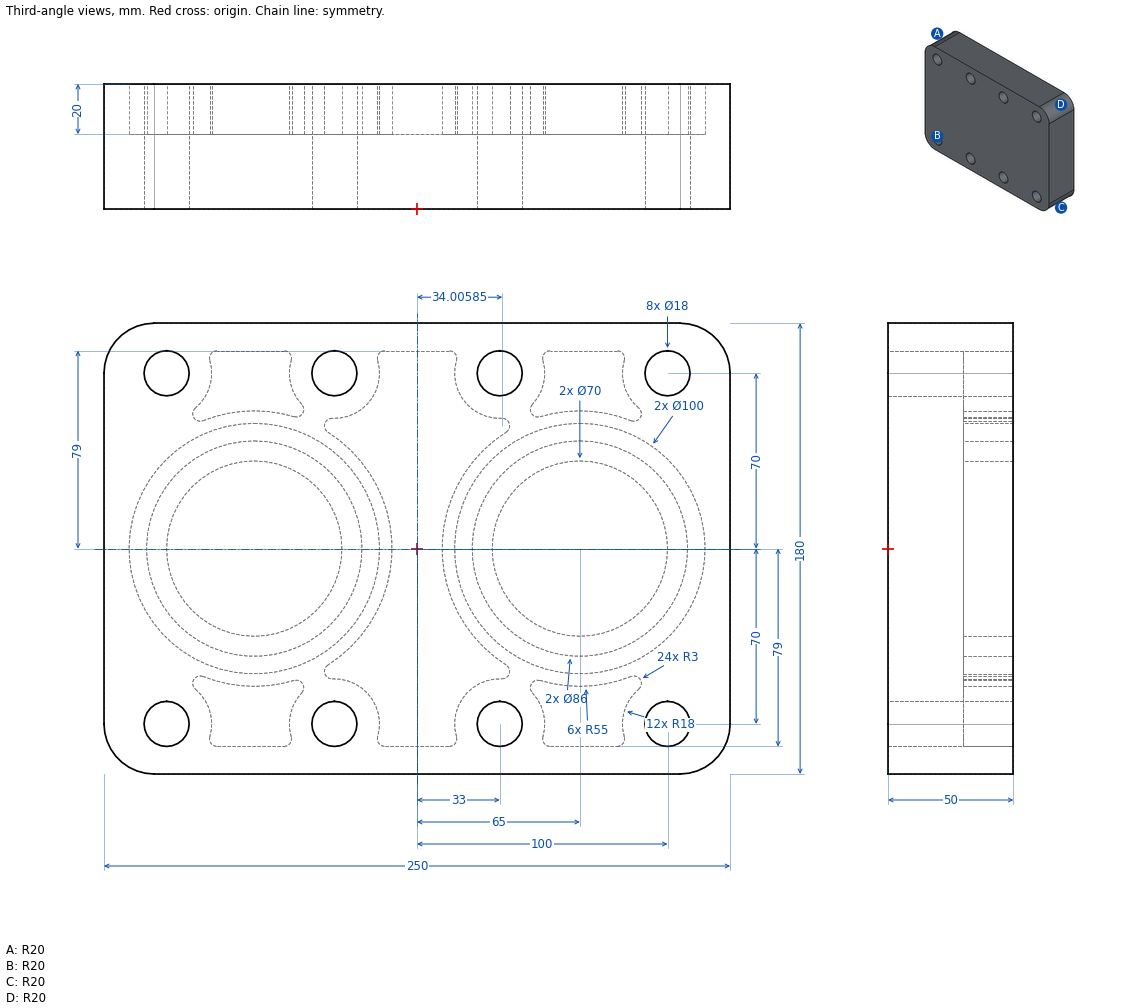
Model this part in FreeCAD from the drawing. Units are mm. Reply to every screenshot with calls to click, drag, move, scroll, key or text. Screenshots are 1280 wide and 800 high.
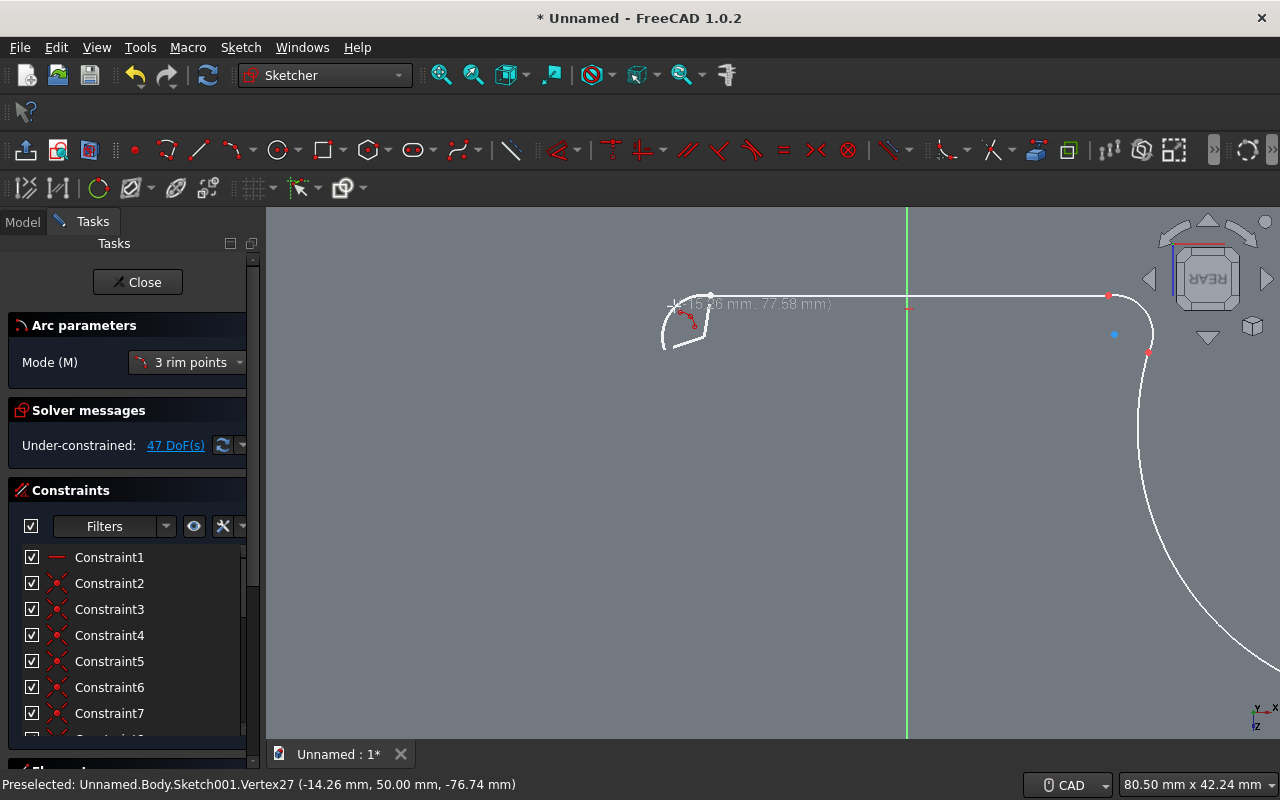
click(672, 306)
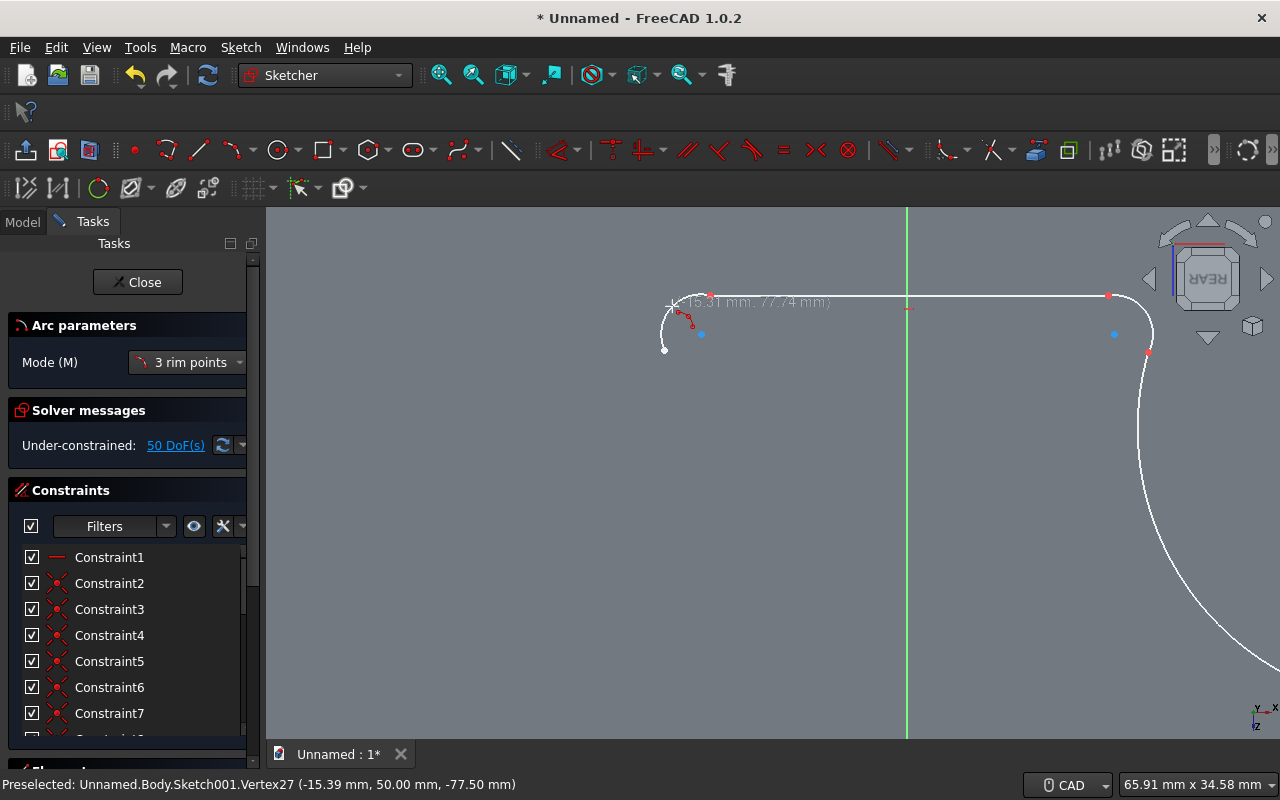
scroll(673, 312, down, 10)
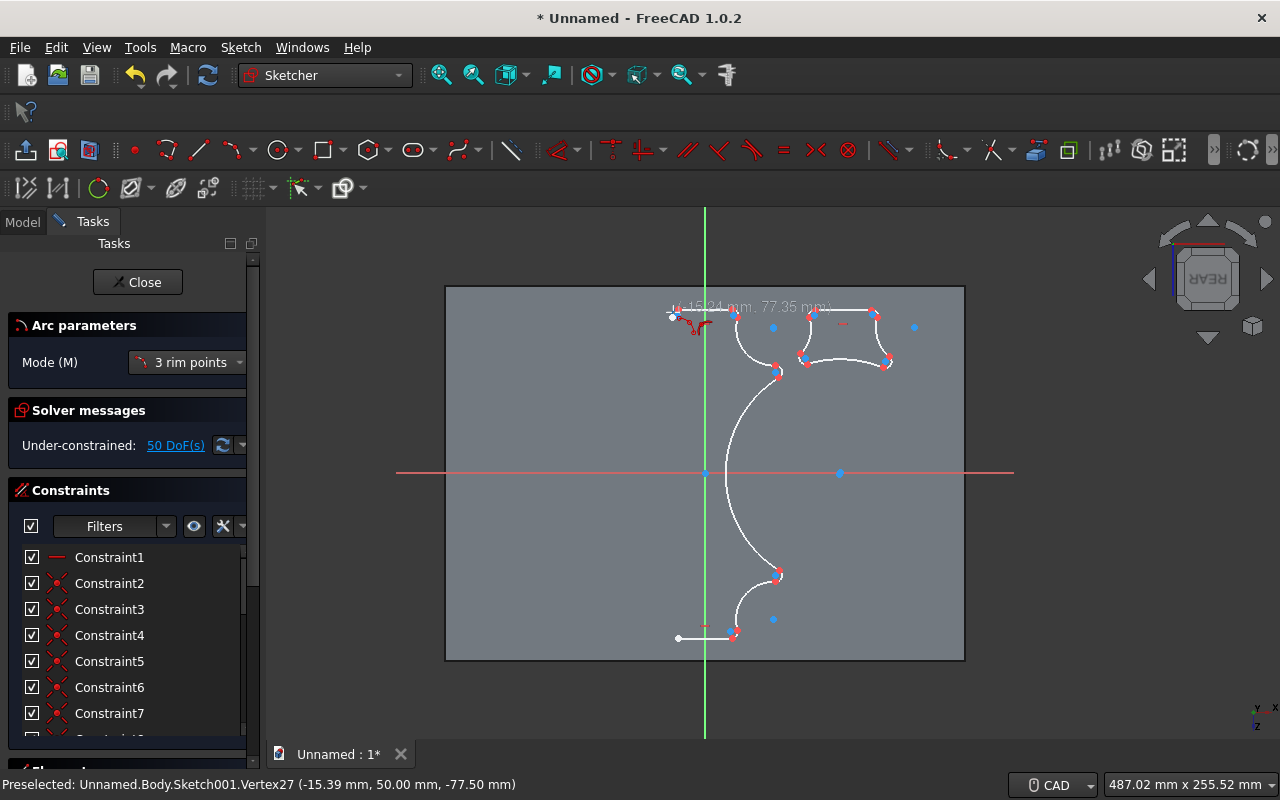
scroll(672, 317, up, 5)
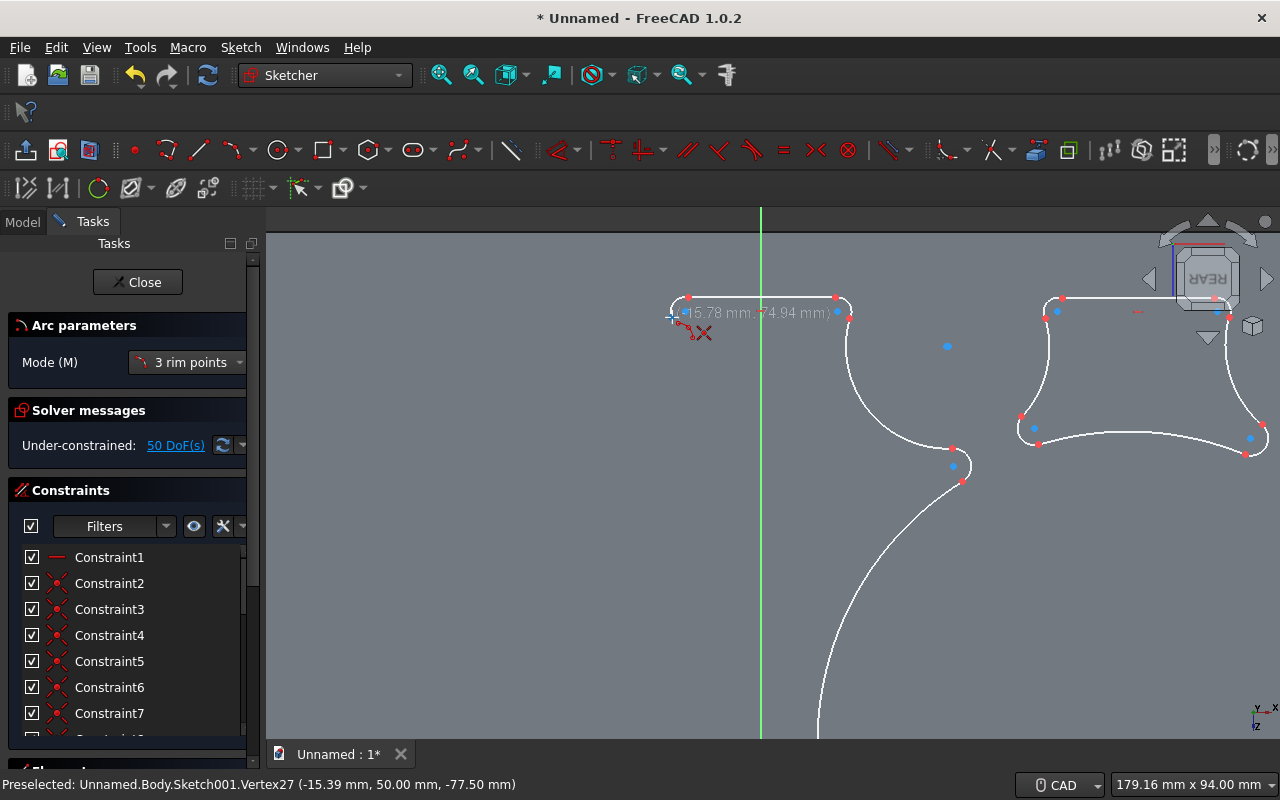
click(672, 318)
click(570, 447)
click(655, 408)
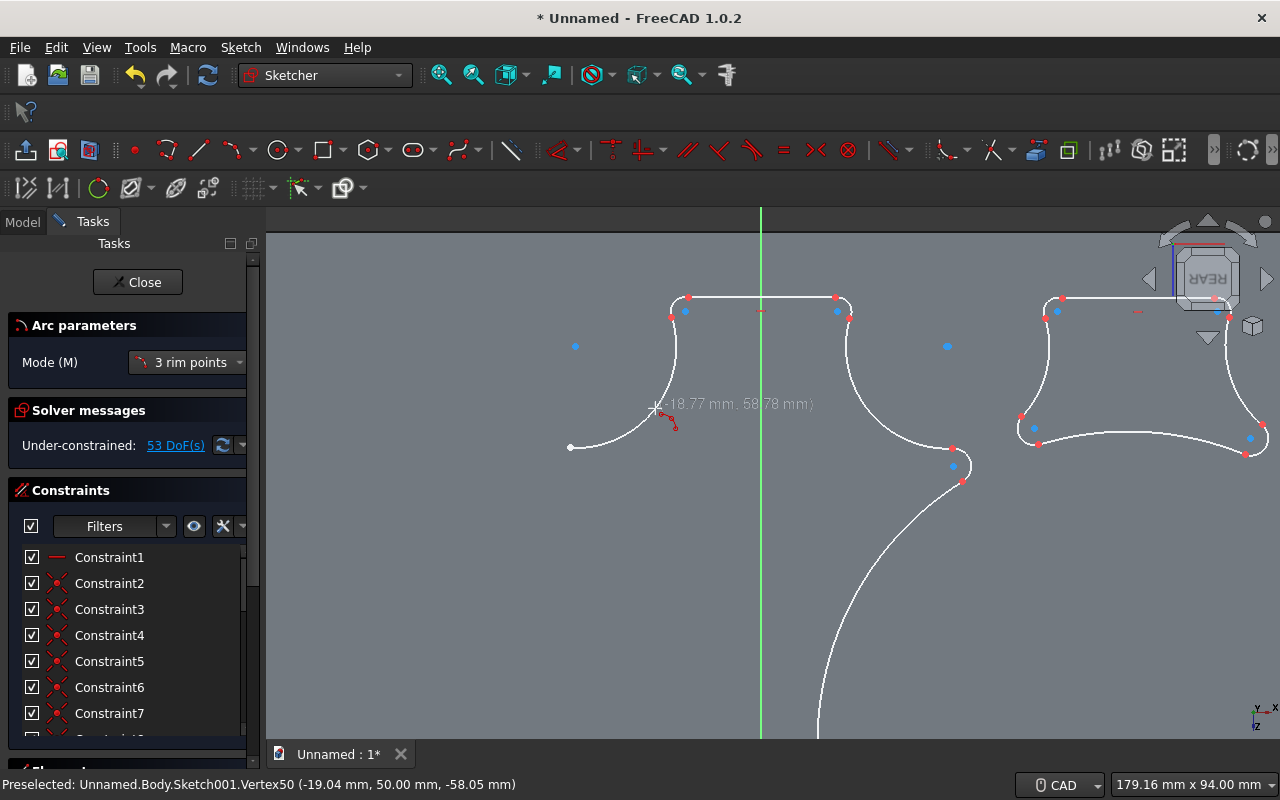
click(570, 448)
click(560, 479)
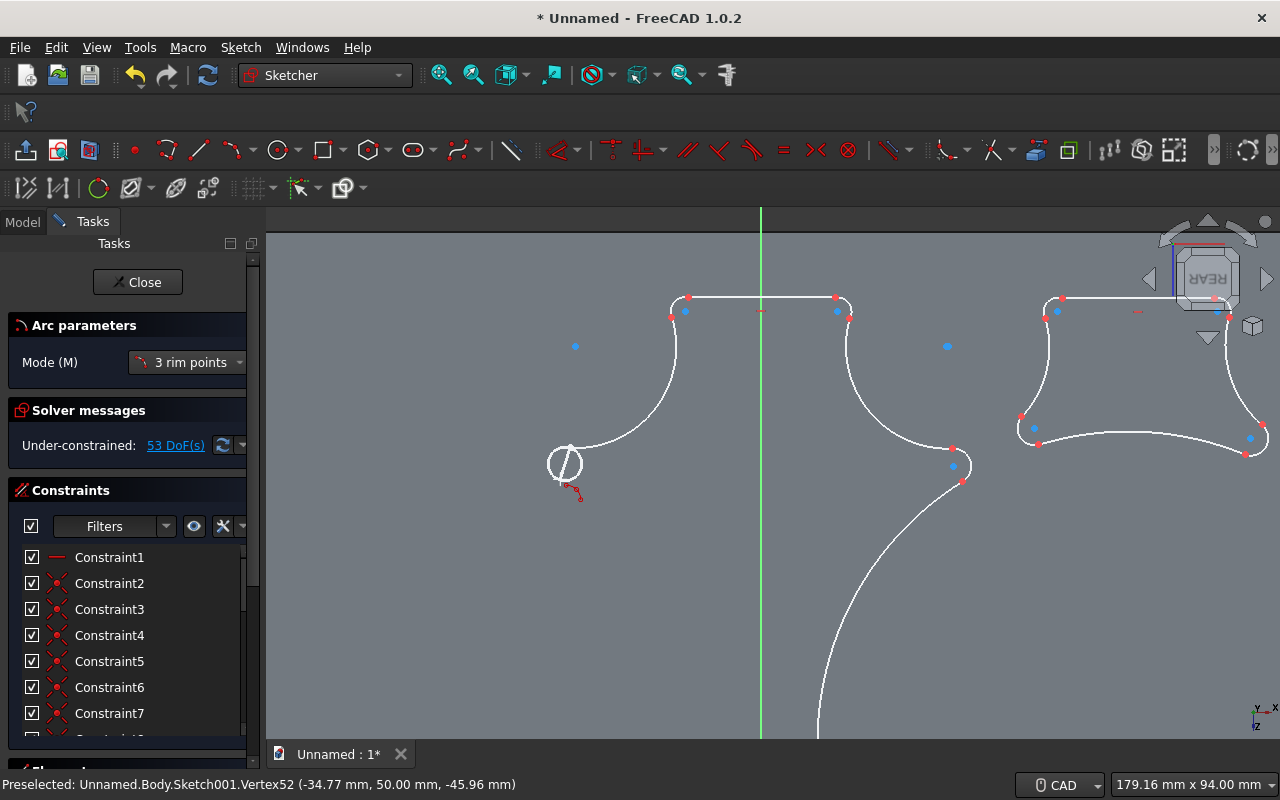
scroll(553, 459, up, 2)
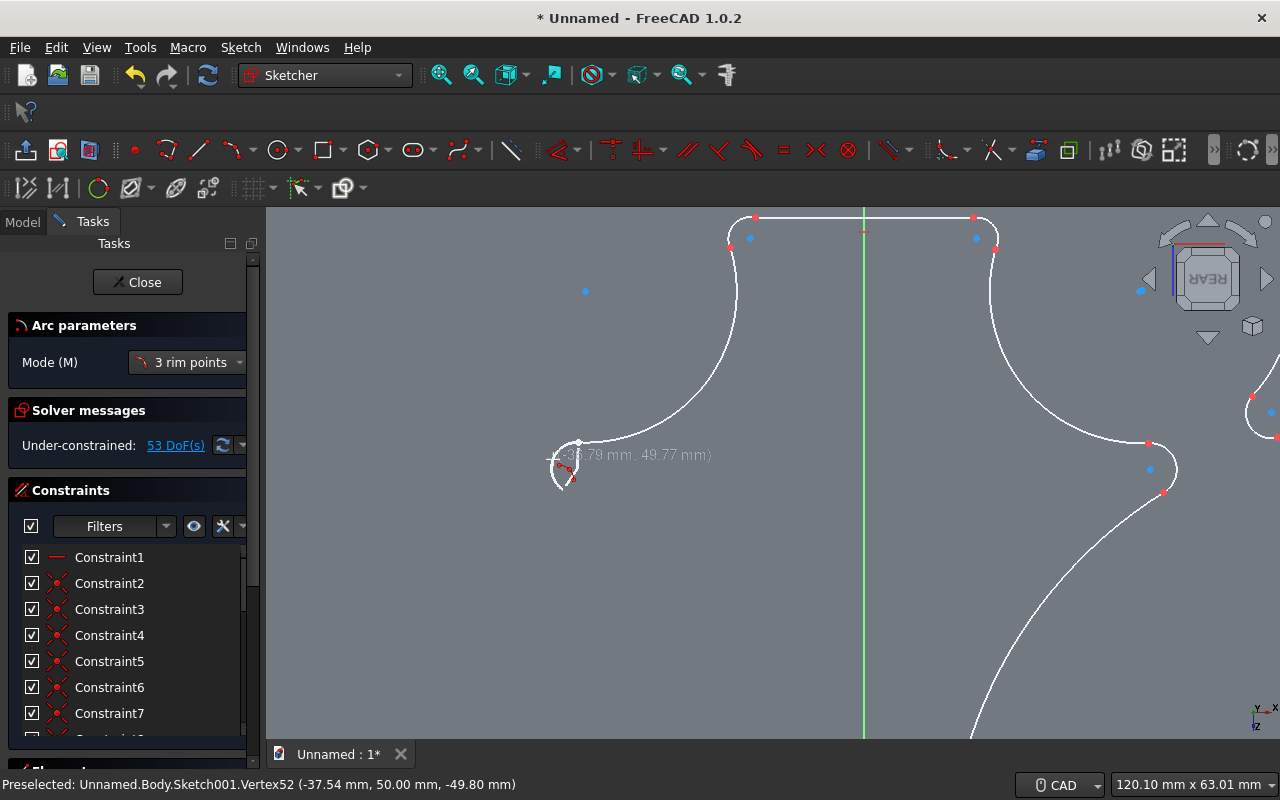
click(552, 459)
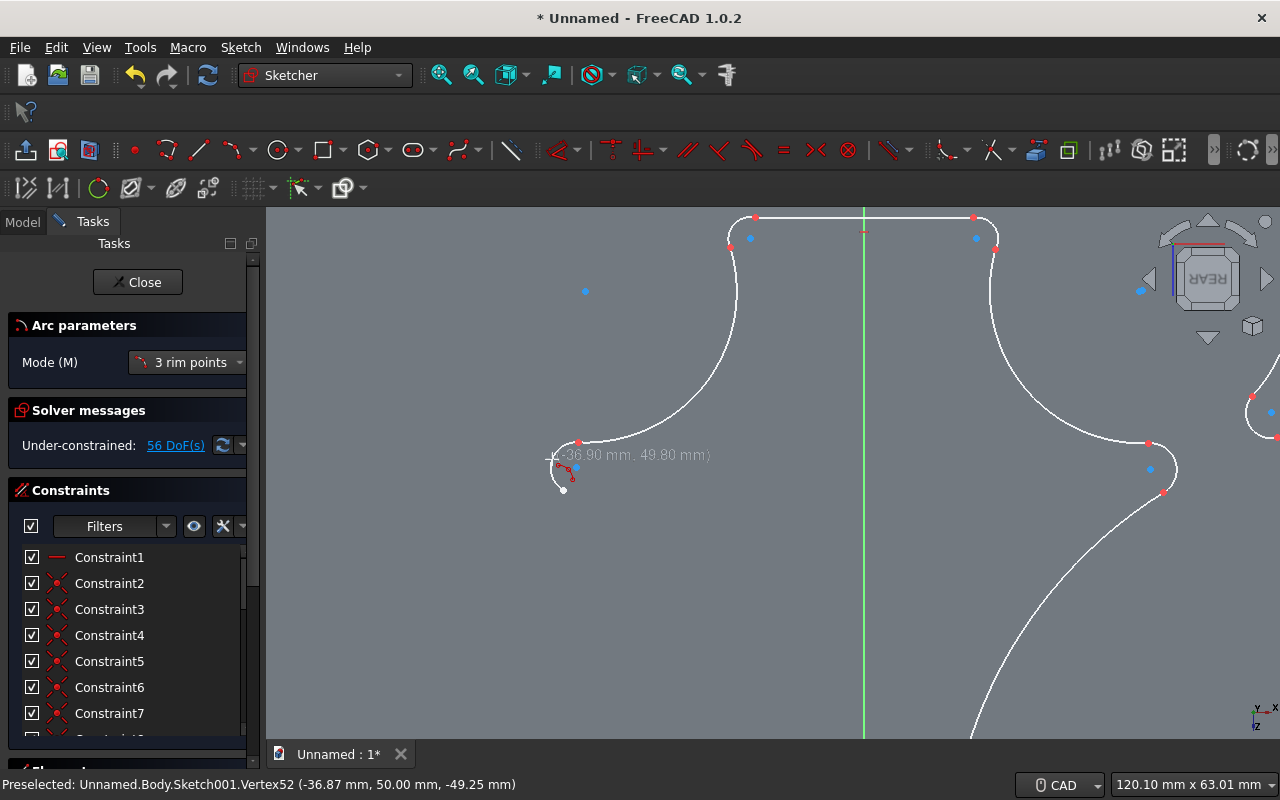
click(563, 490)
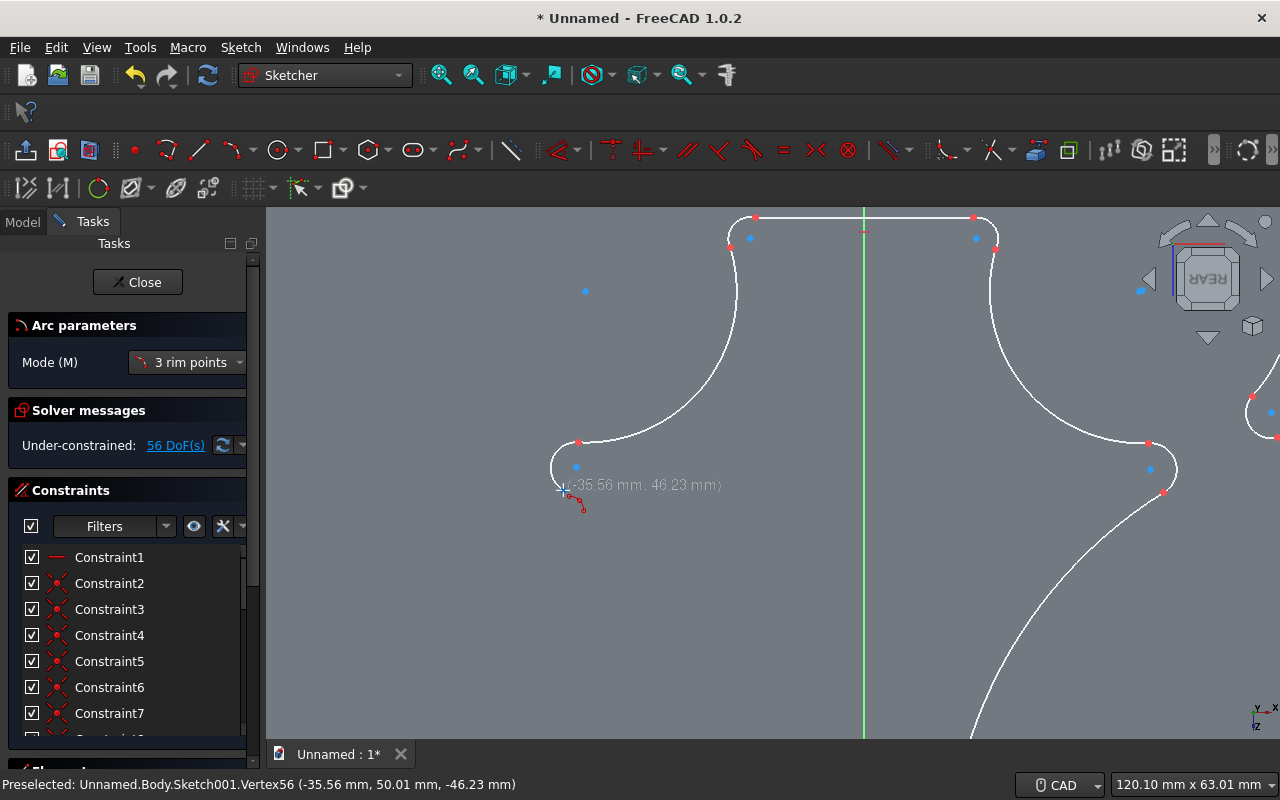
scroll(652, 340, down, 7)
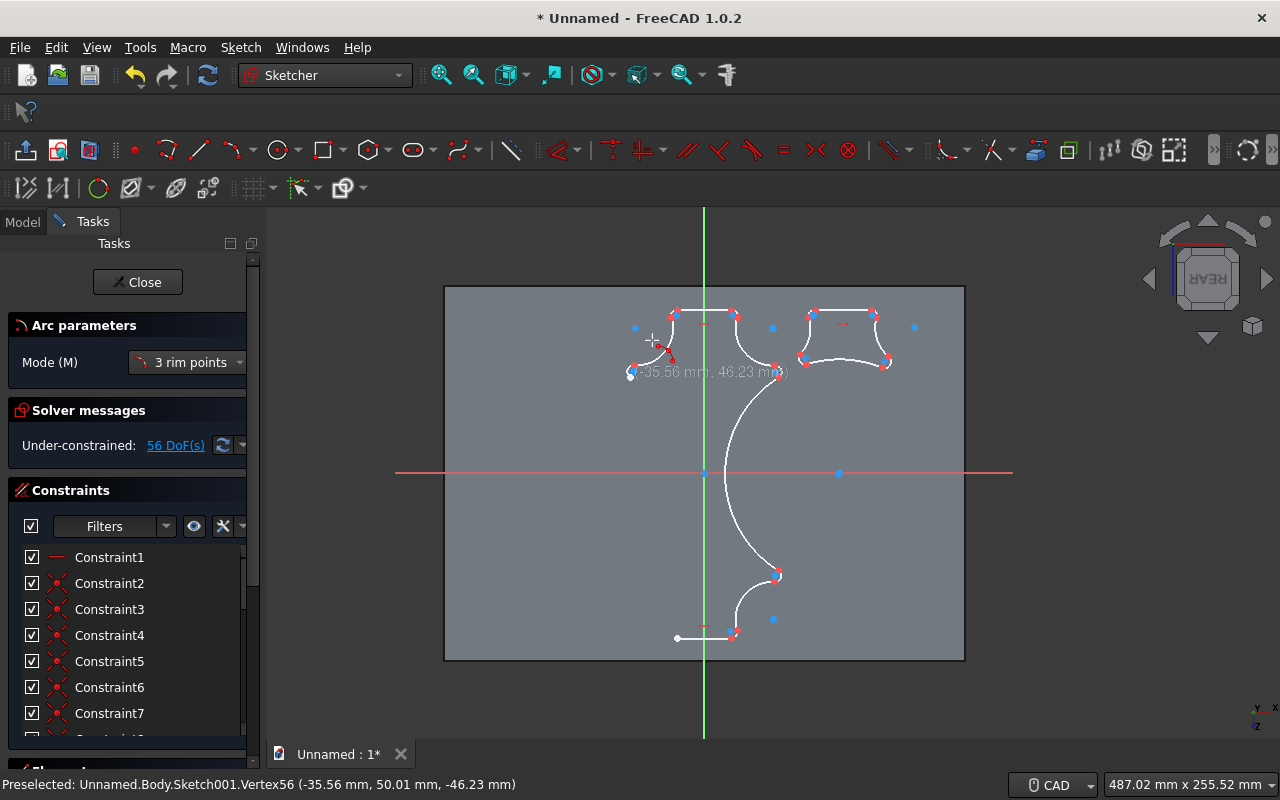
click(630, 570)
click(681, 496)